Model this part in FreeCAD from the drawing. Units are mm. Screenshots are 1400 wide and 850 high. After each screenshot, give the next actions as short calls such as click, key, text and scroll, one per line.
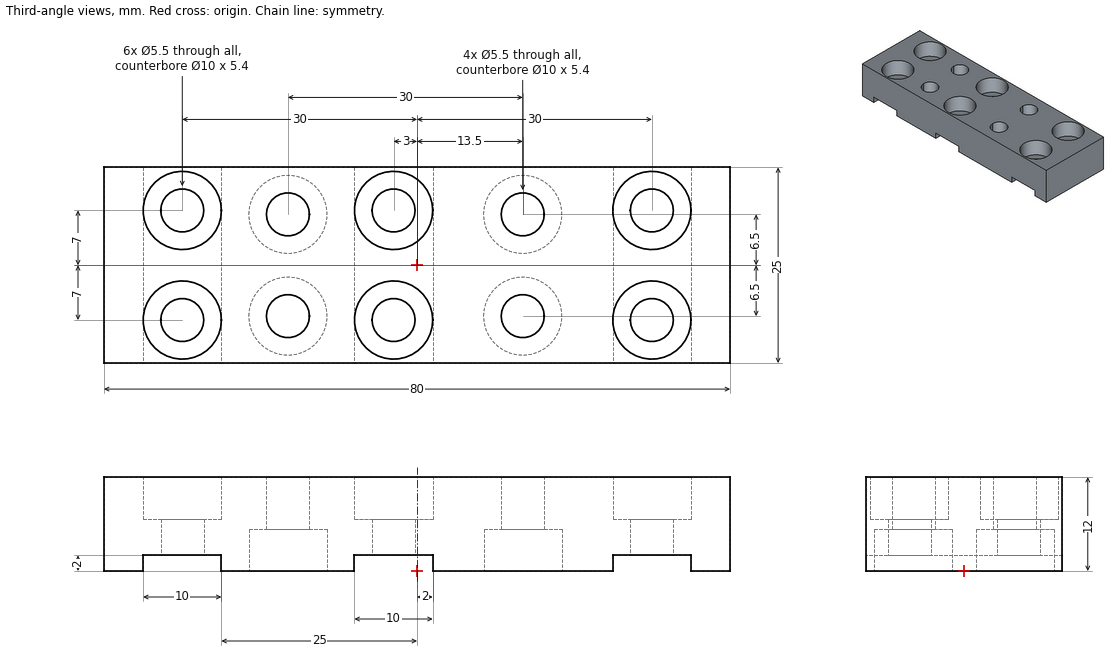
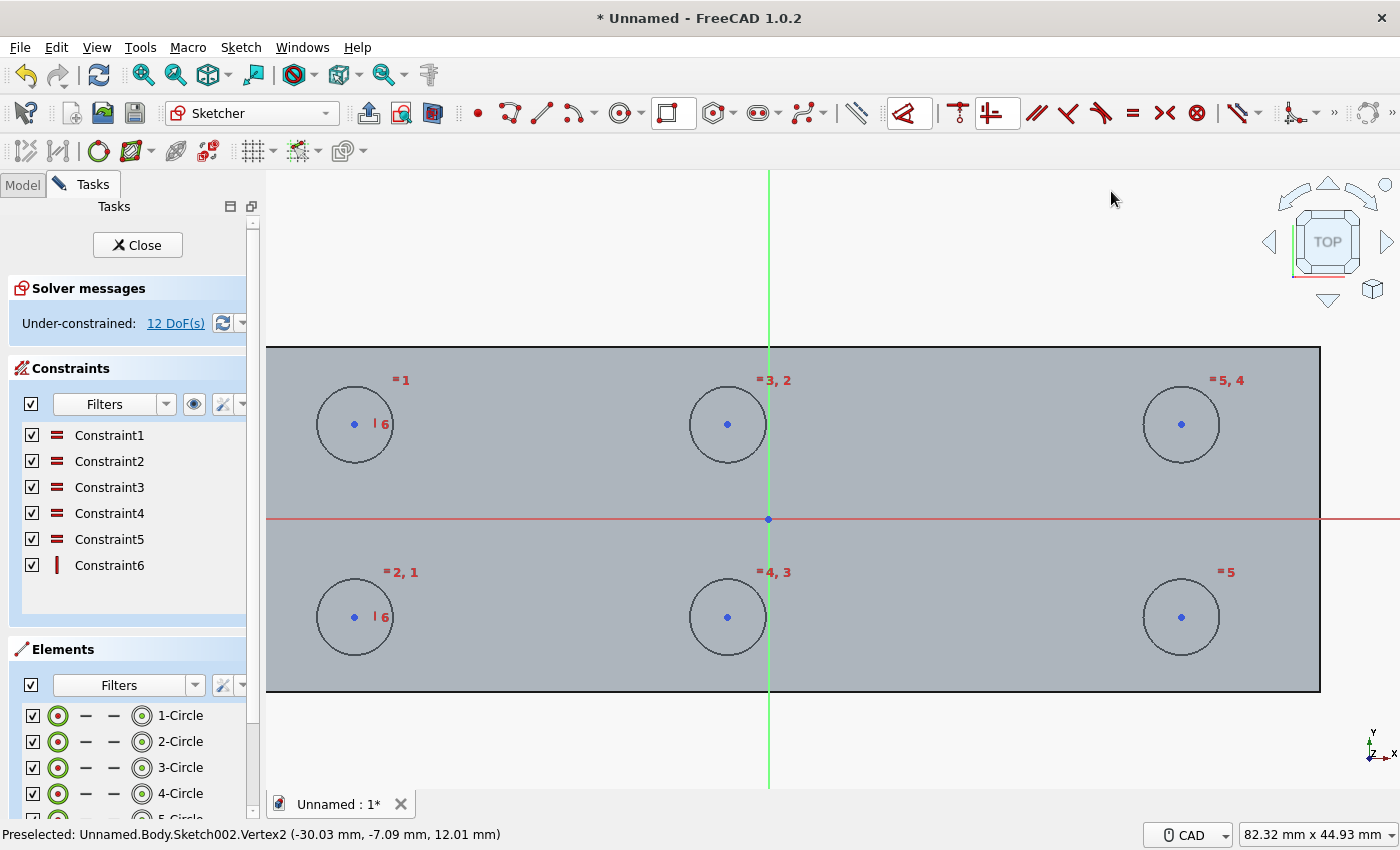
click(355, 425)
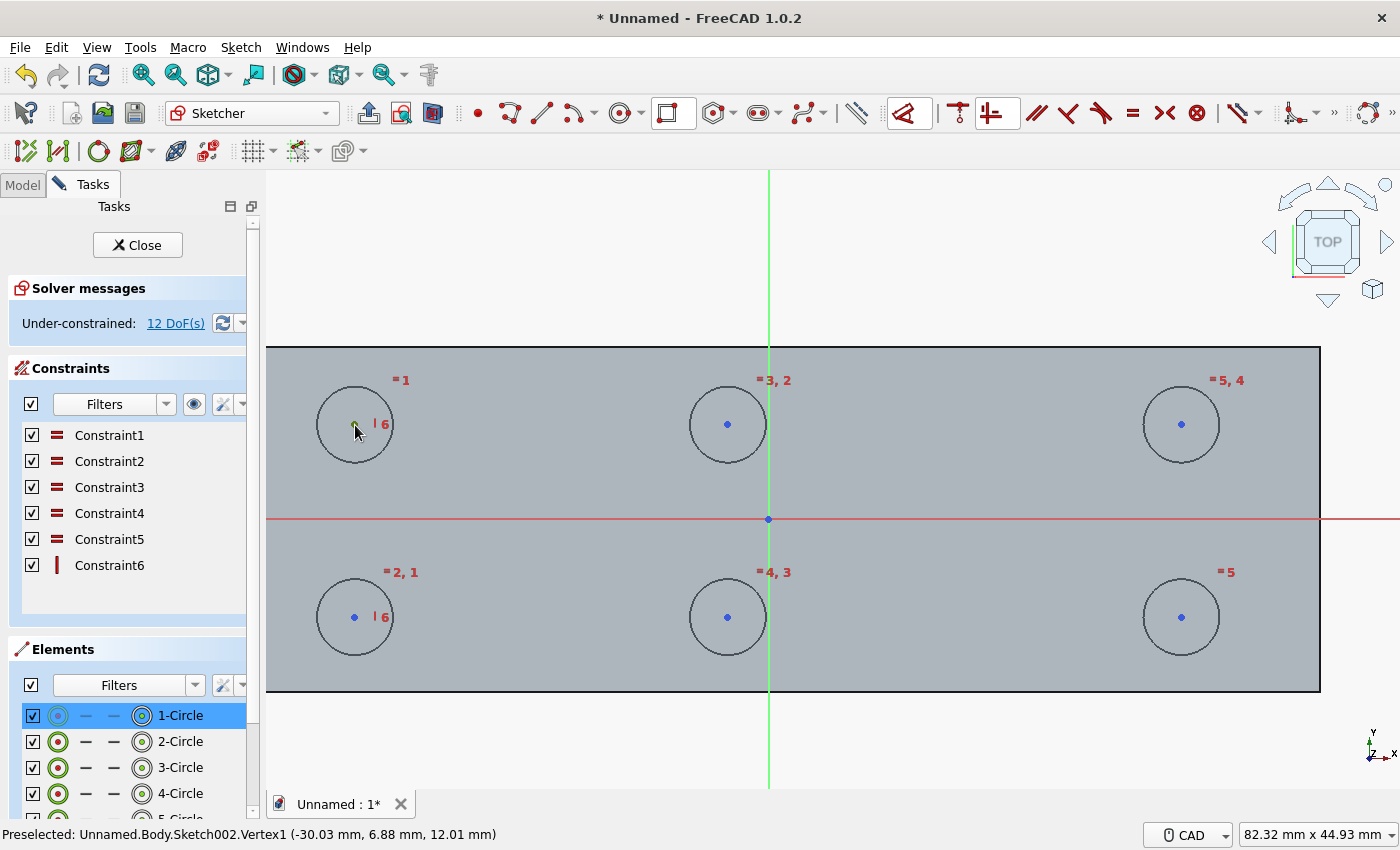
click(728, 425)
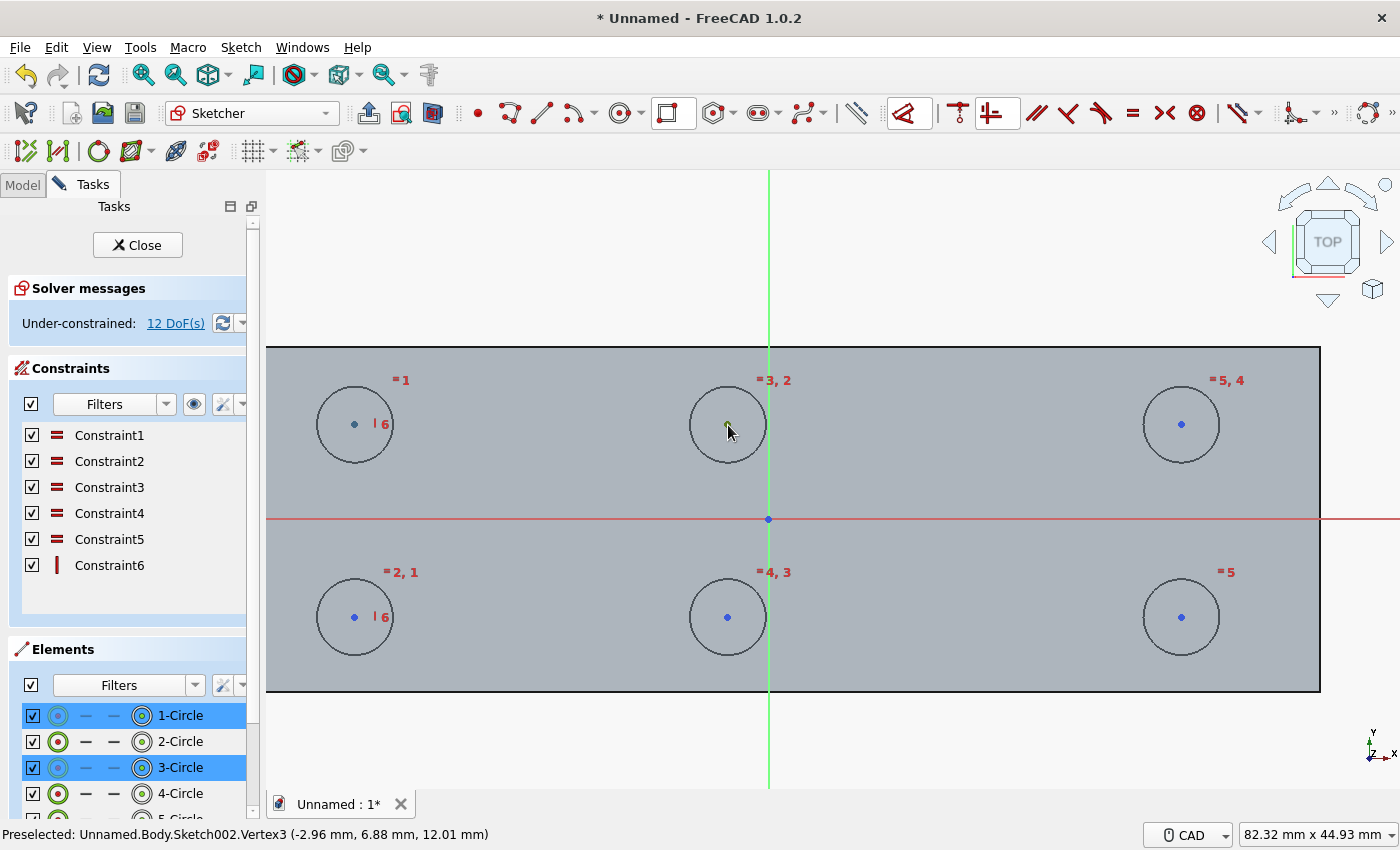
key(h)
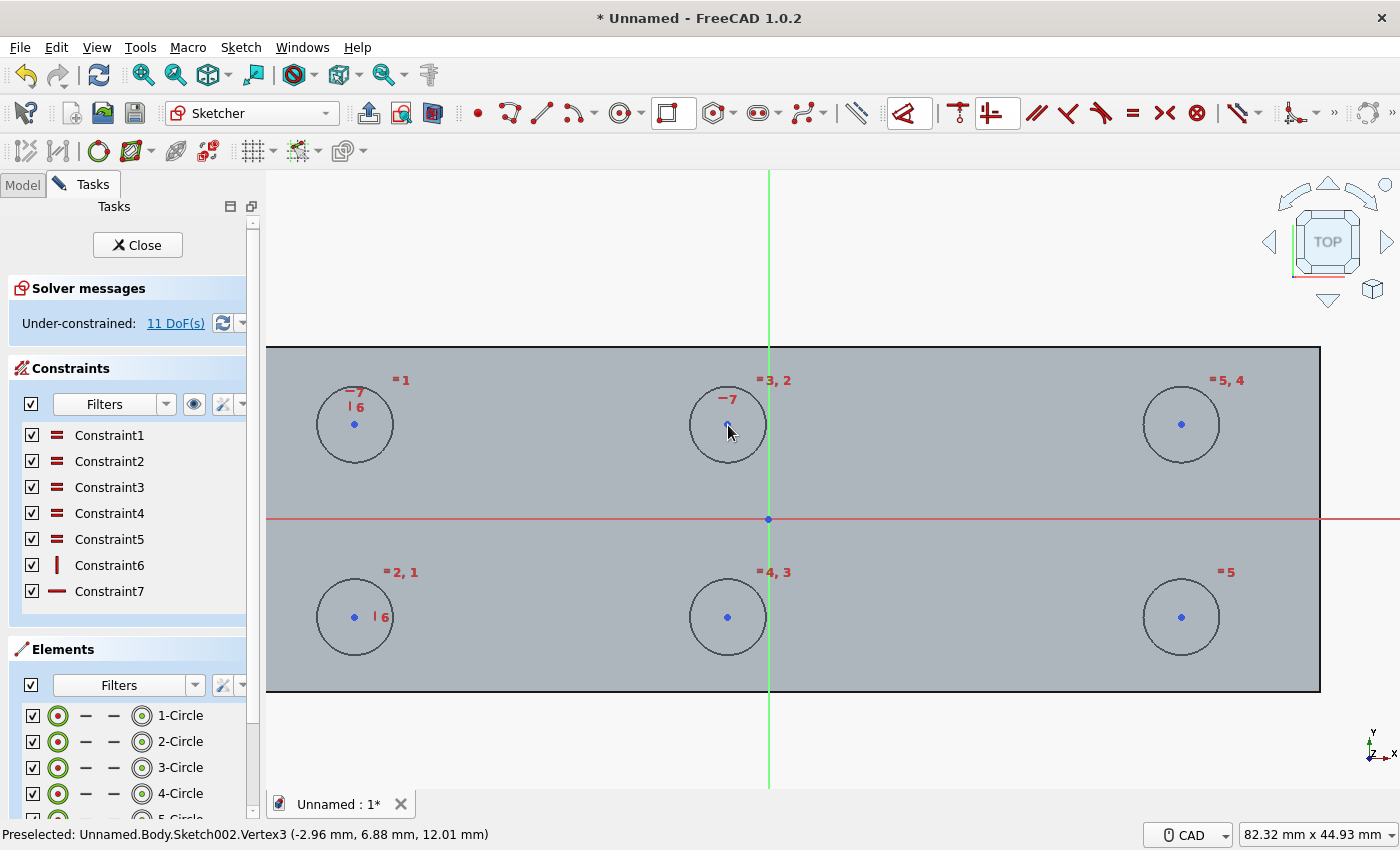
click(728, 425)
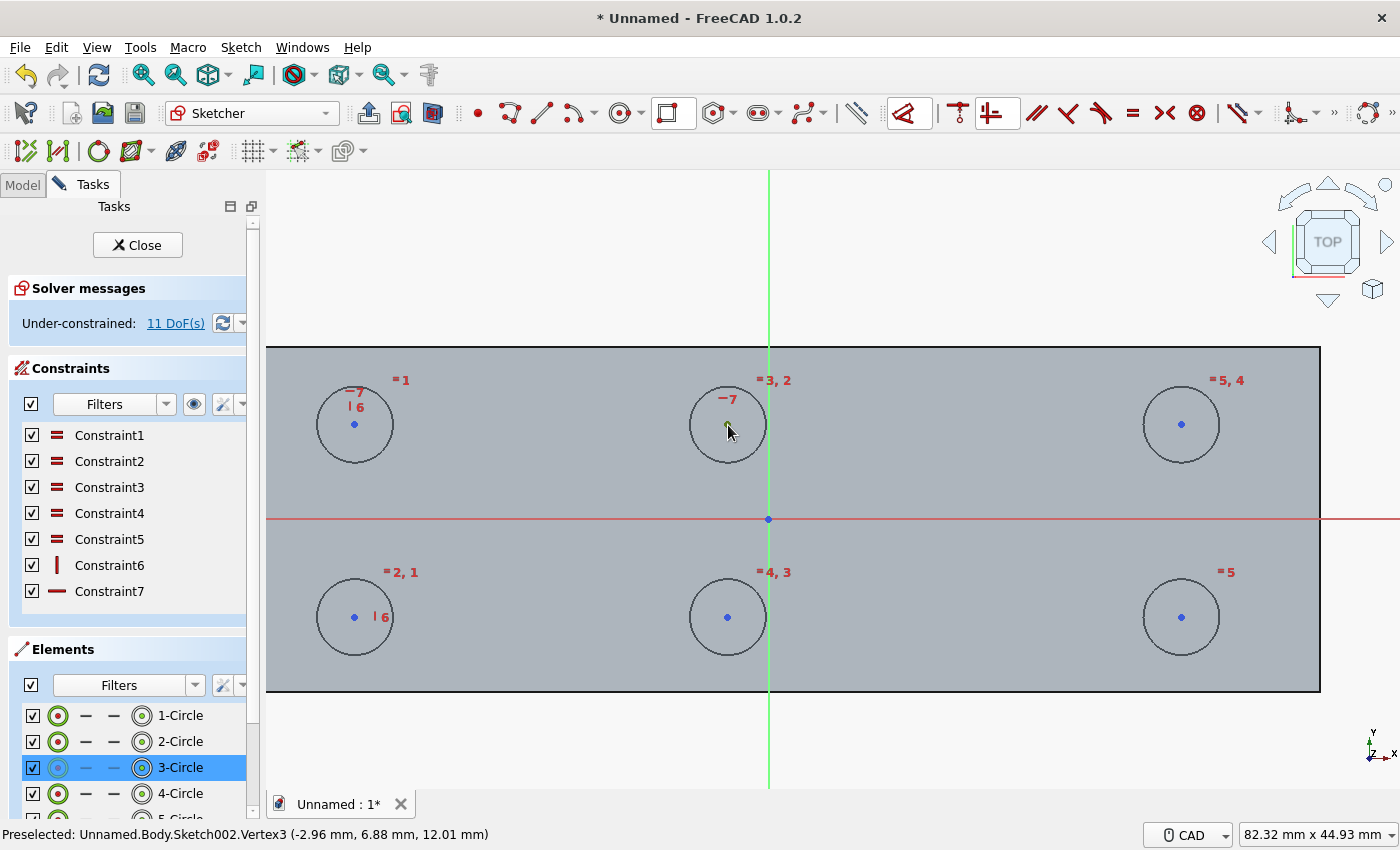
click(728, 617)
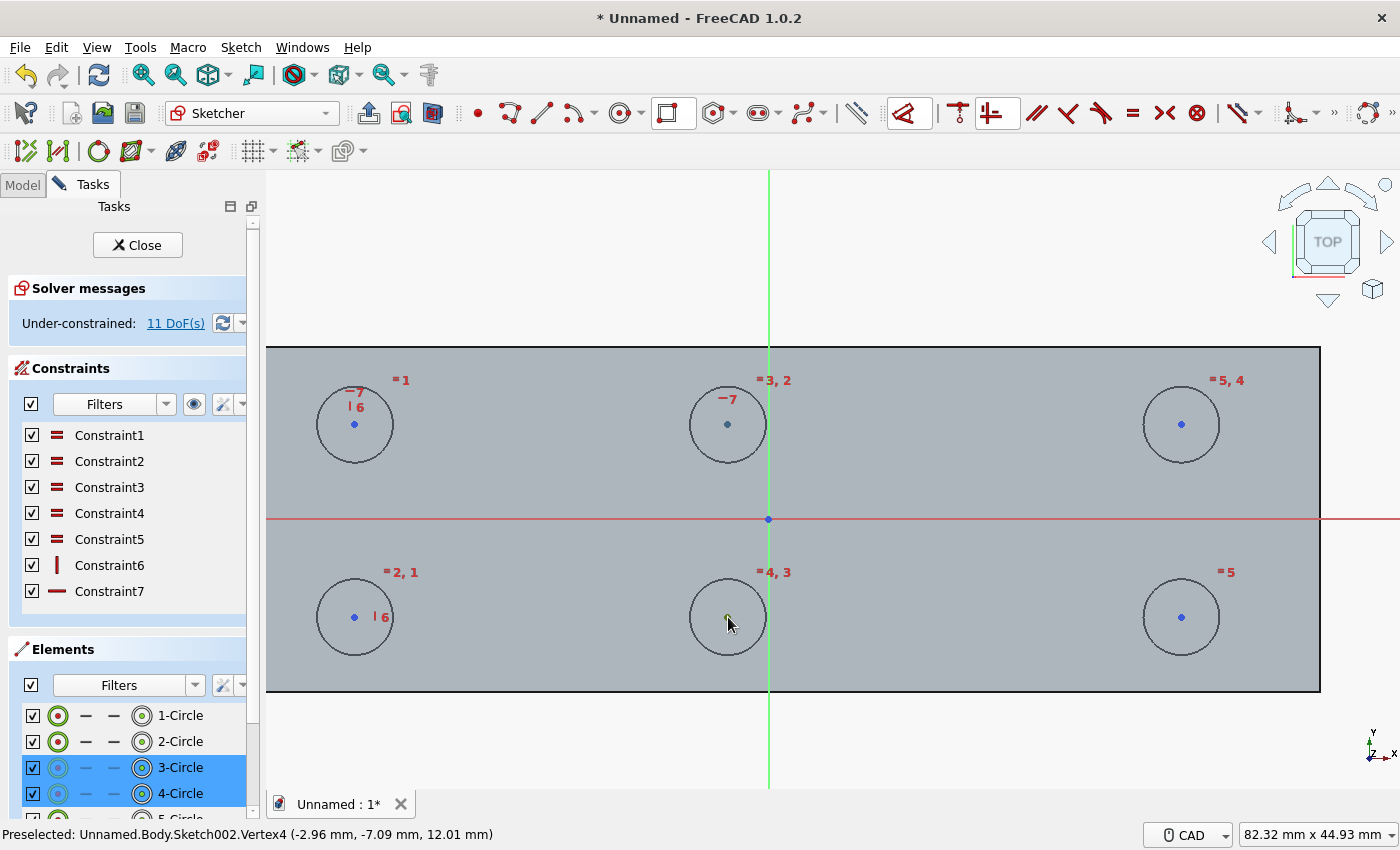
click(1014, 114)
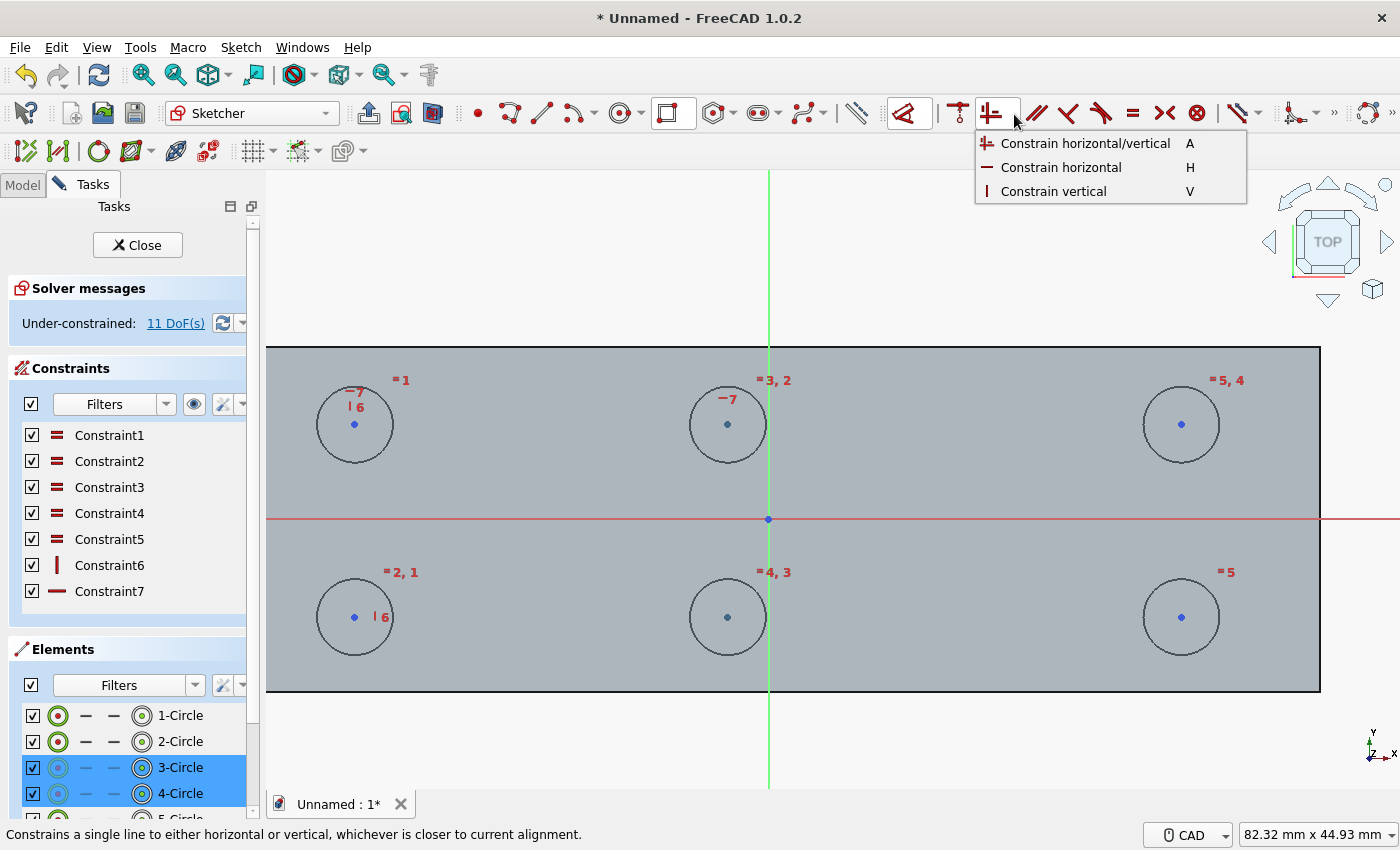
click(1111, 191)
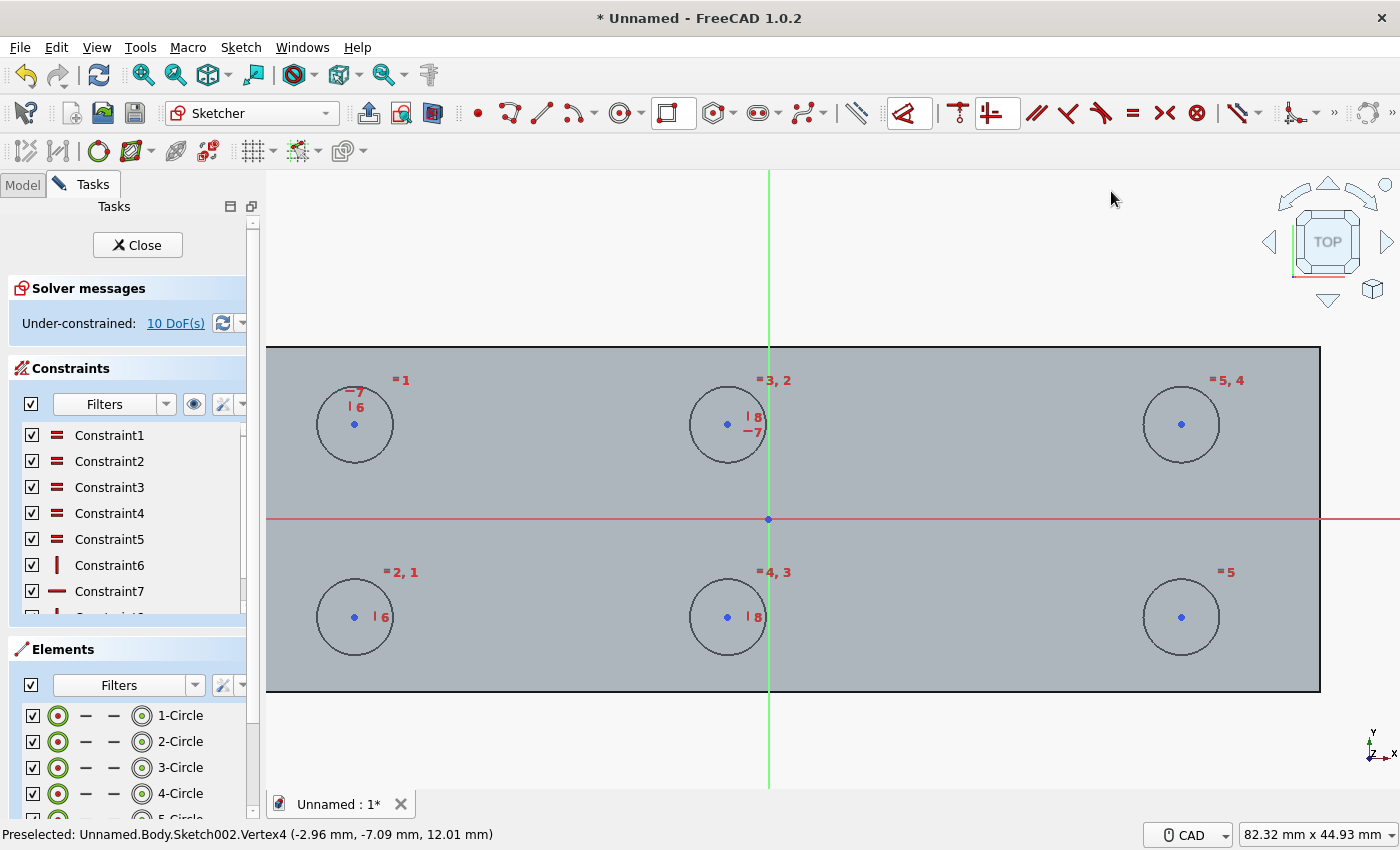
click(355, 617)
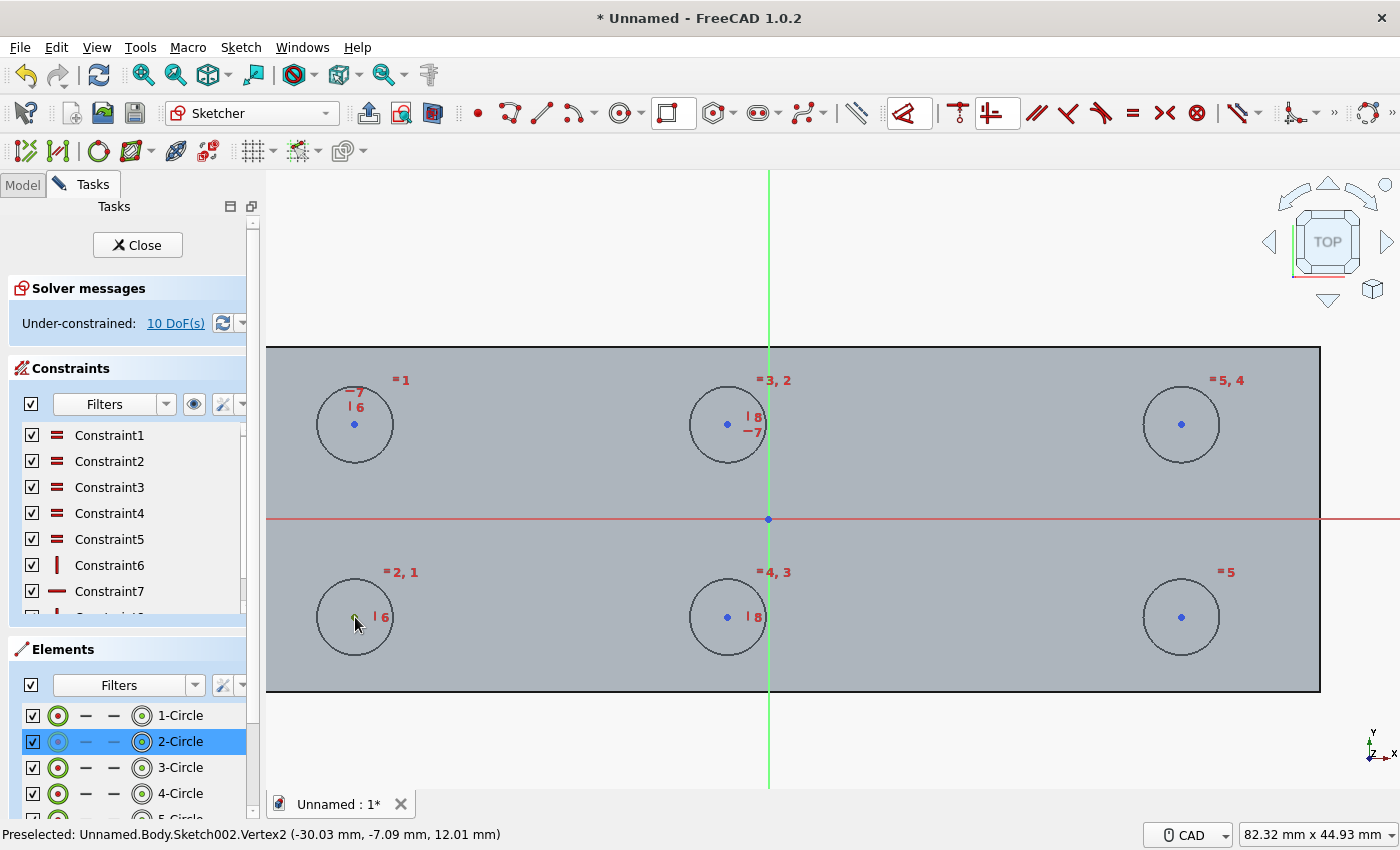
click(728, 617)